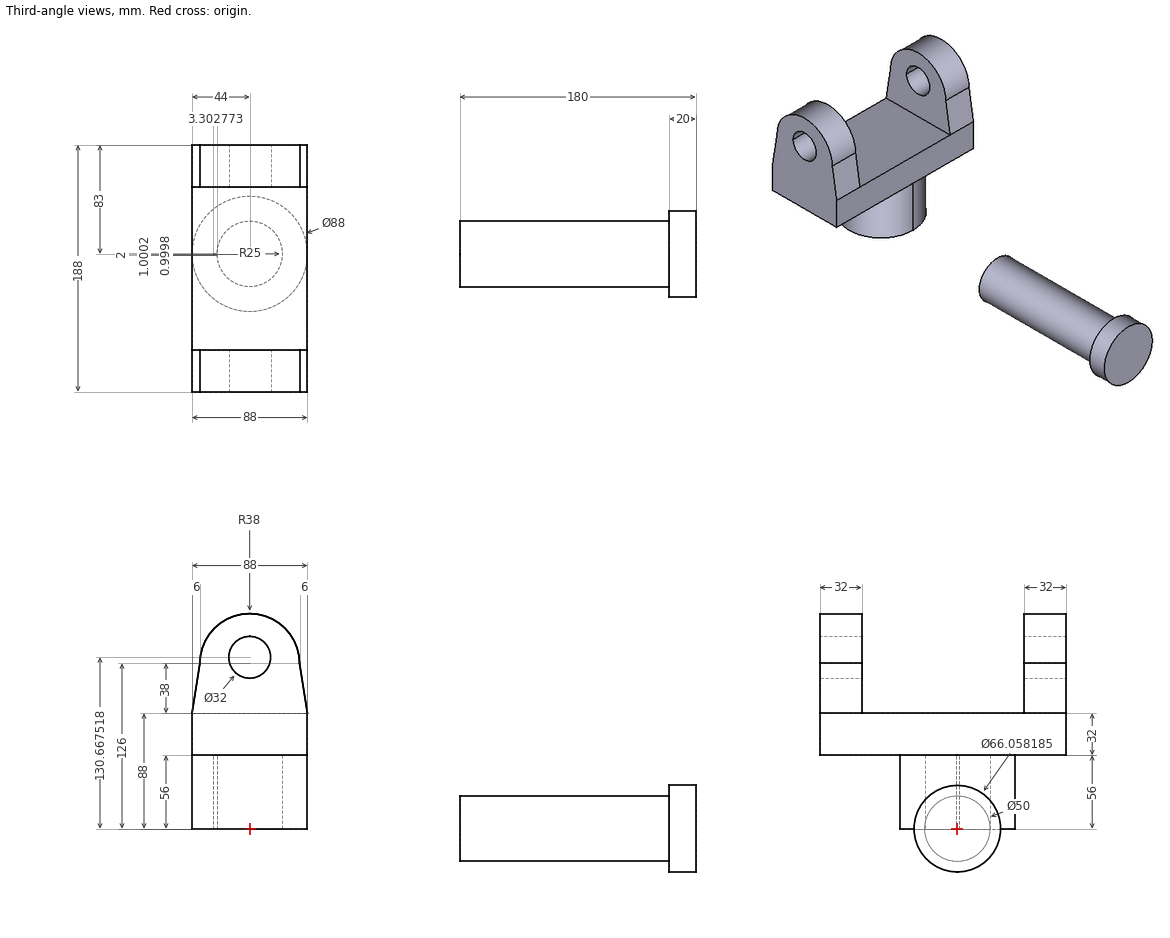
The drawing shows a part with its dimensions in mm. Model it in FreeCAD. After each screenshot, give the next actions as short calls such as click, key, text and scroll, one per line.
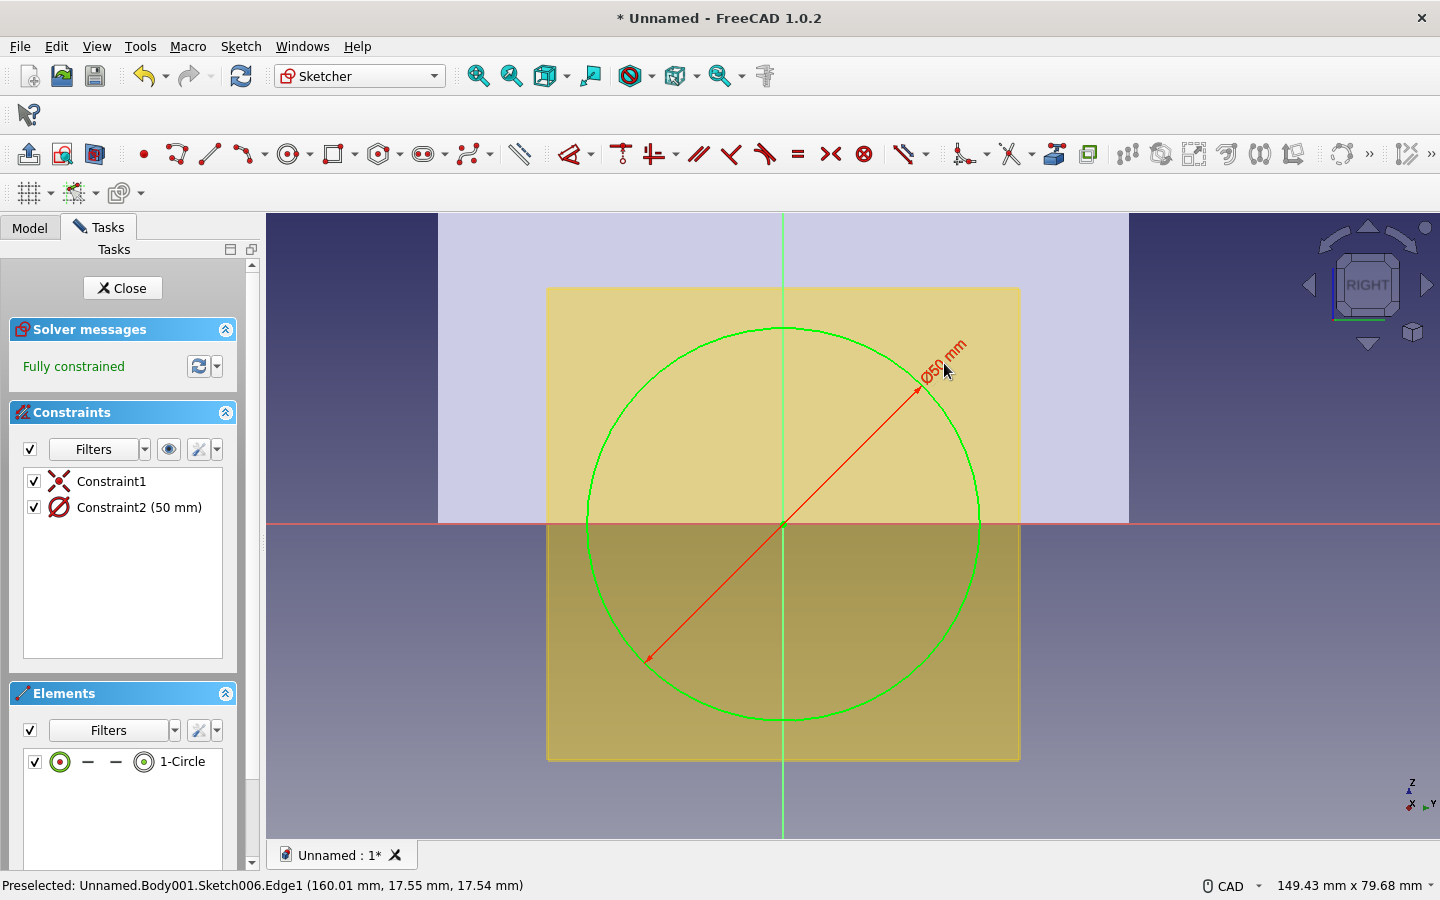
click(123, 288)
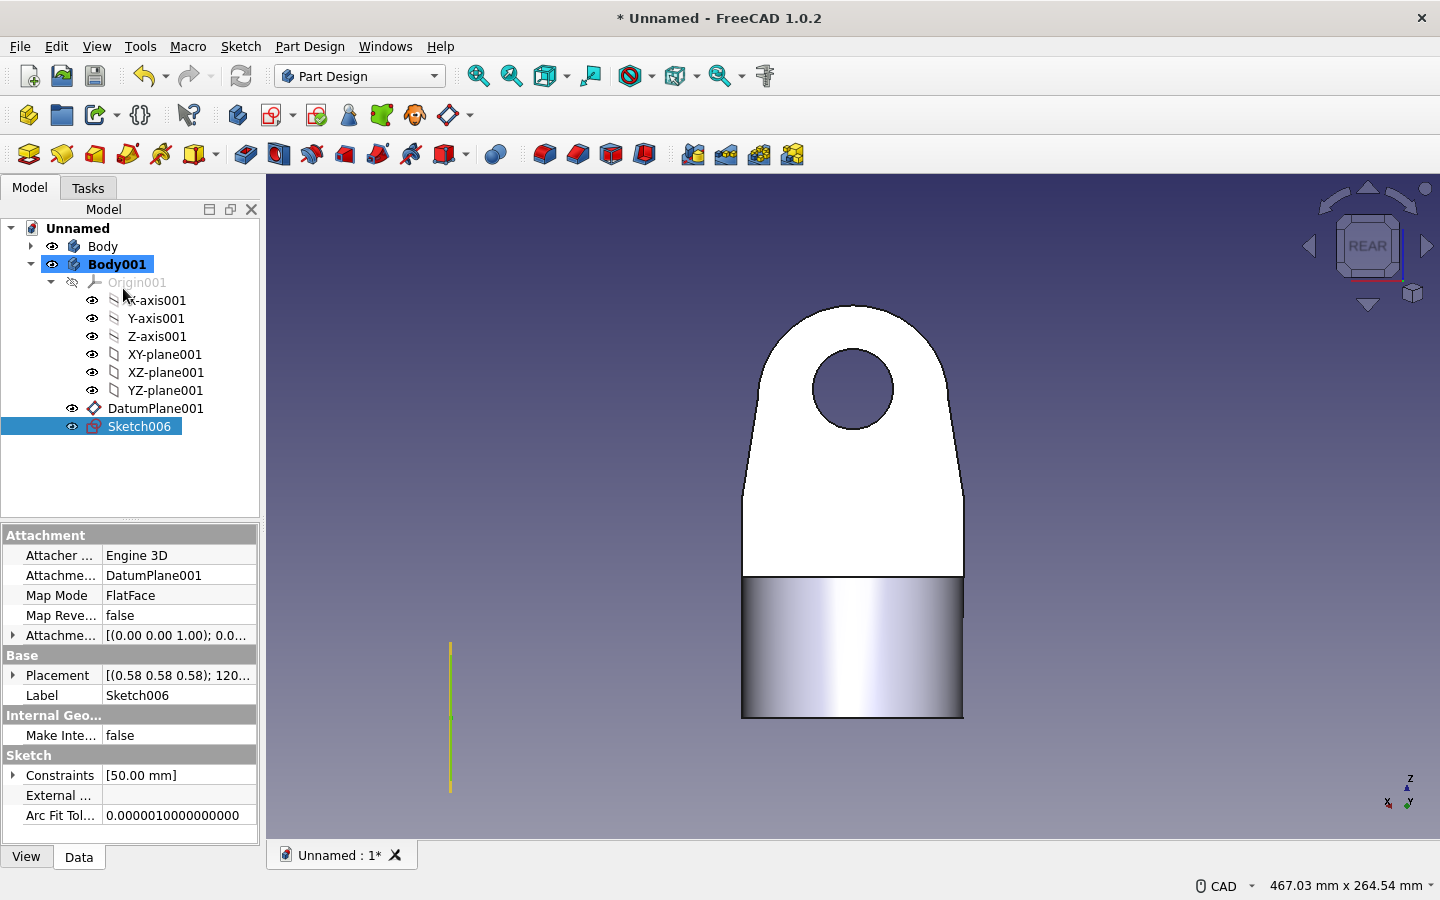
click(29, 154)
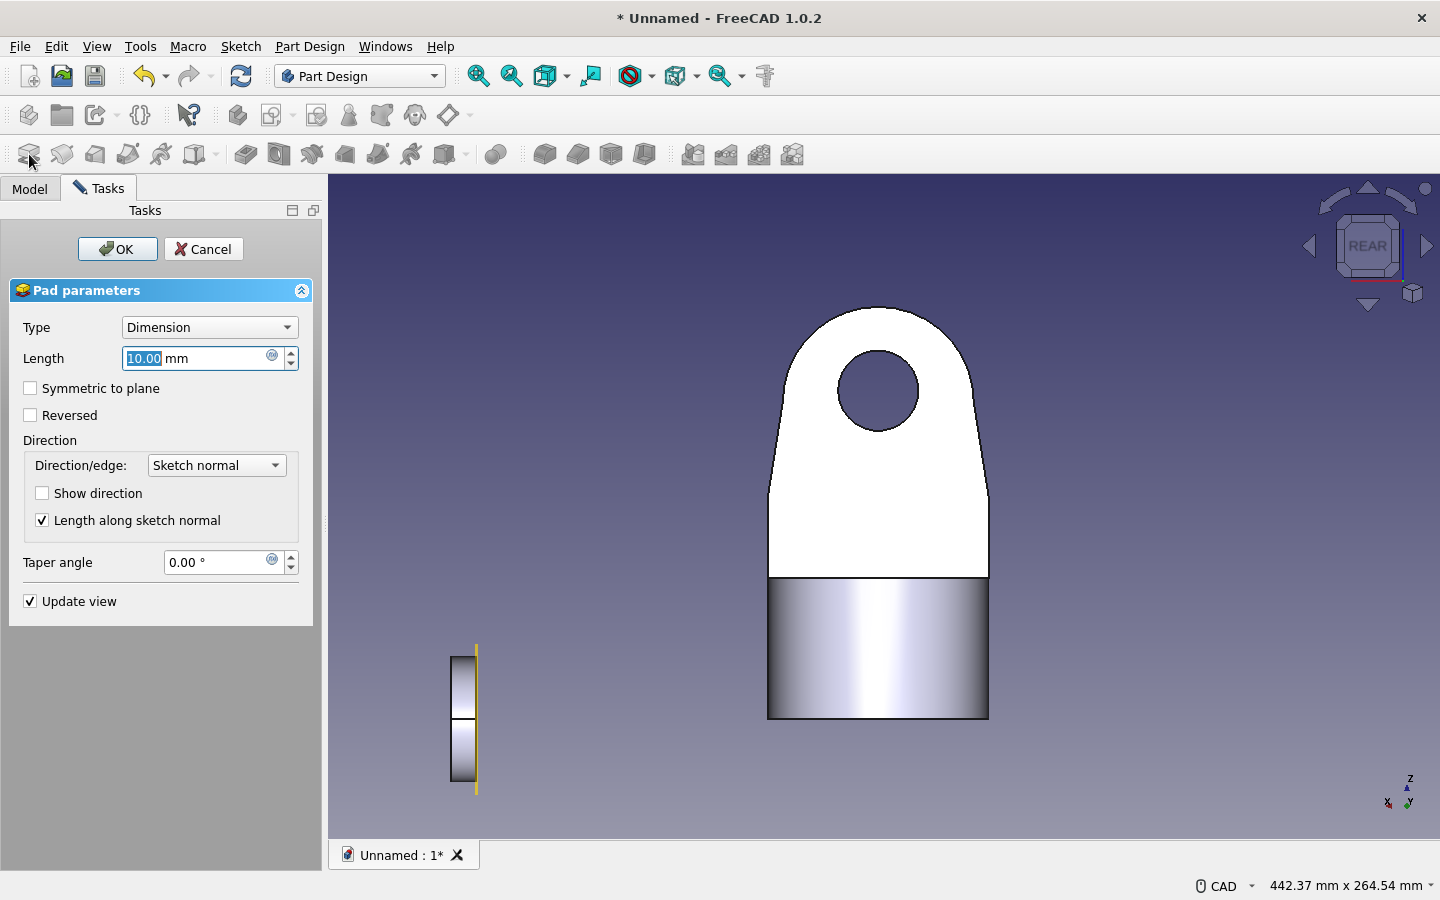
text(180)
key(Tab)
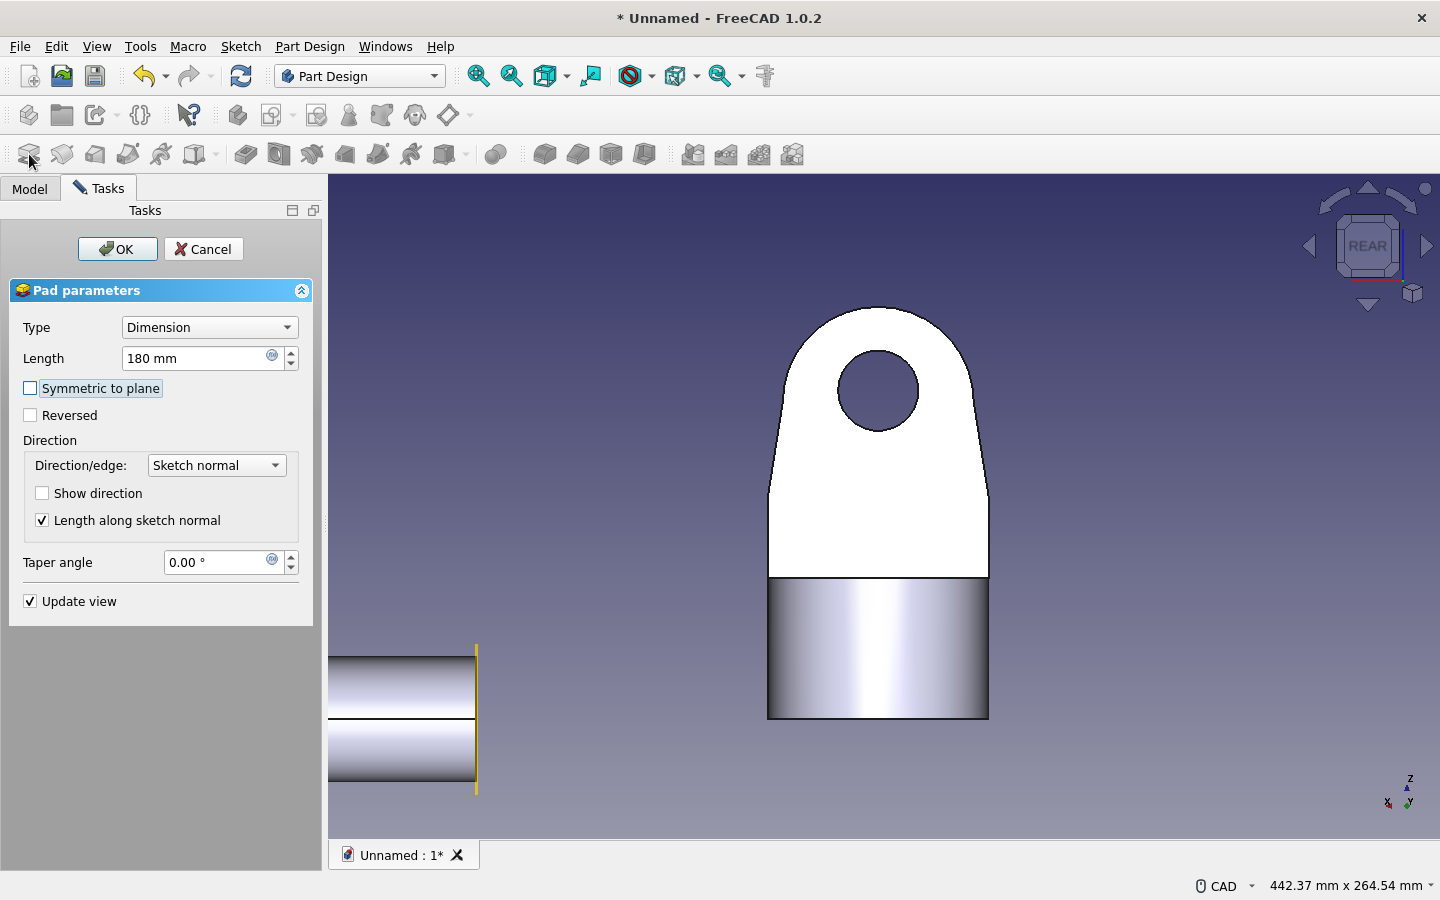
click(118, 249)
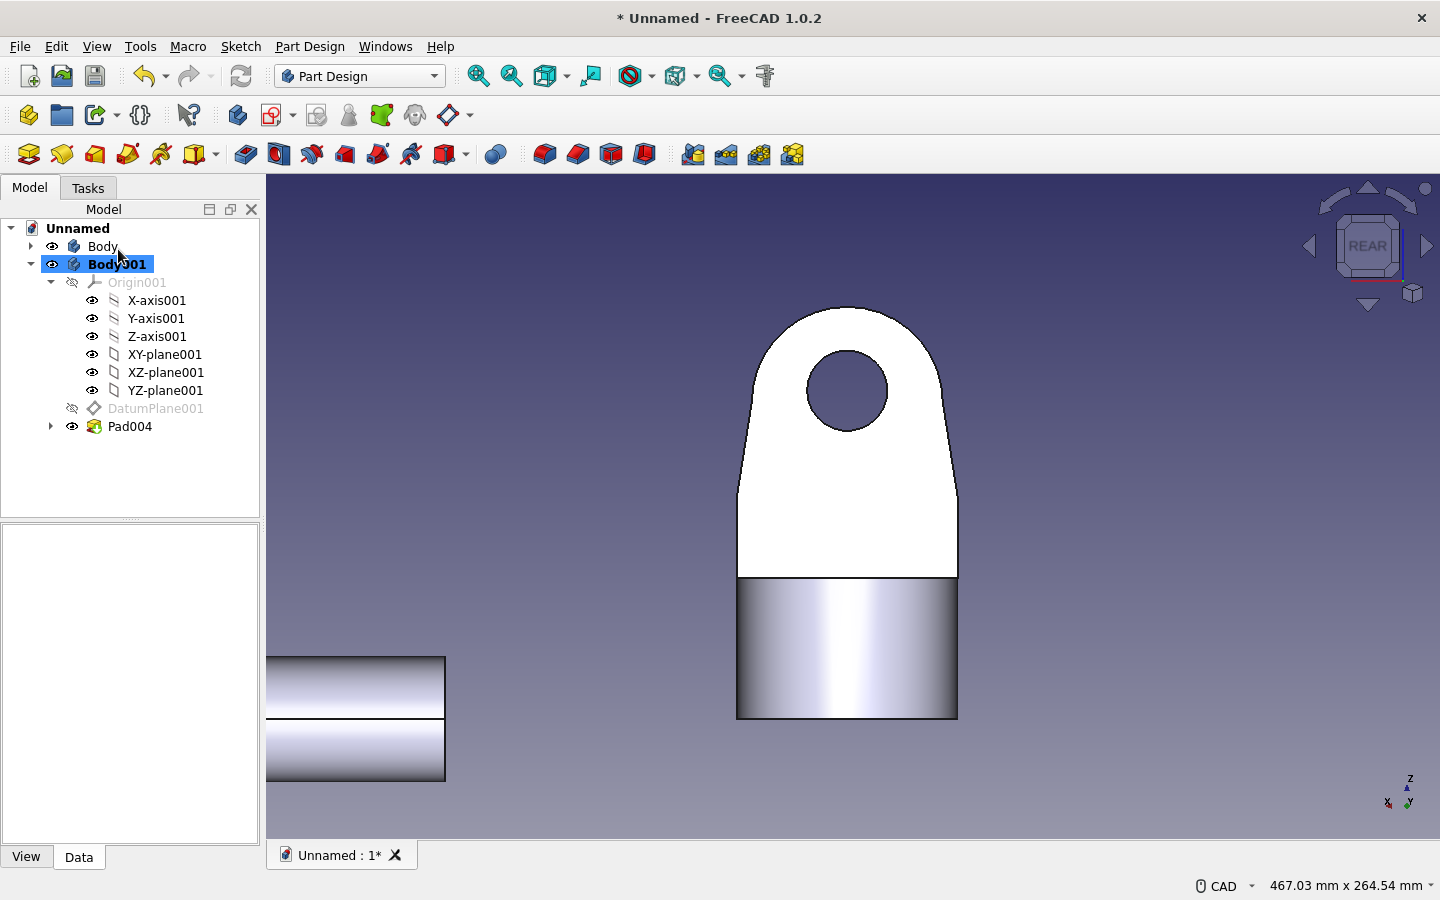
key(v)
key(f)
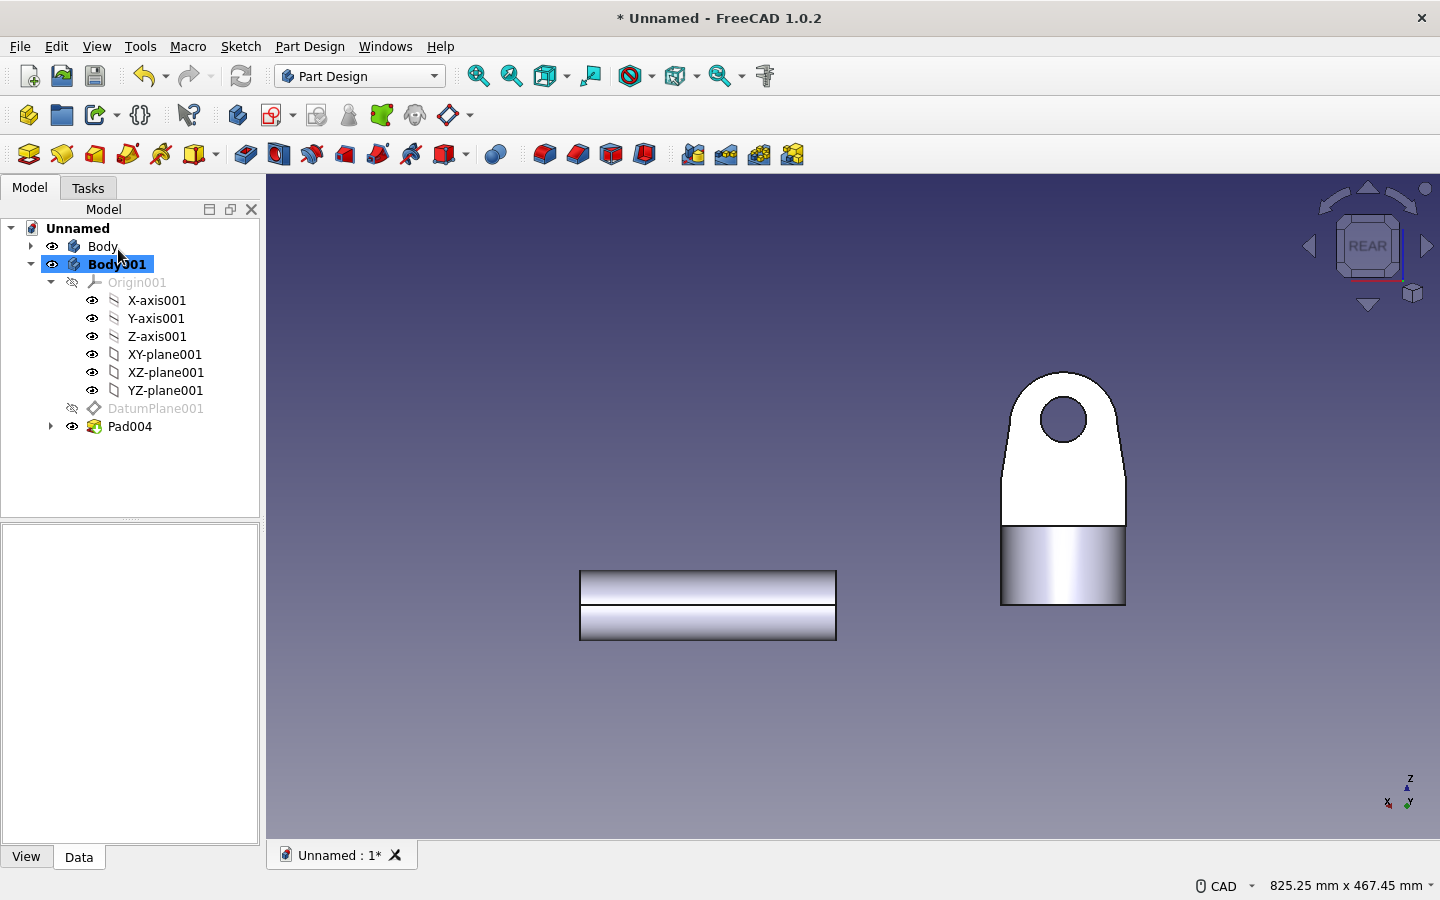
key(0)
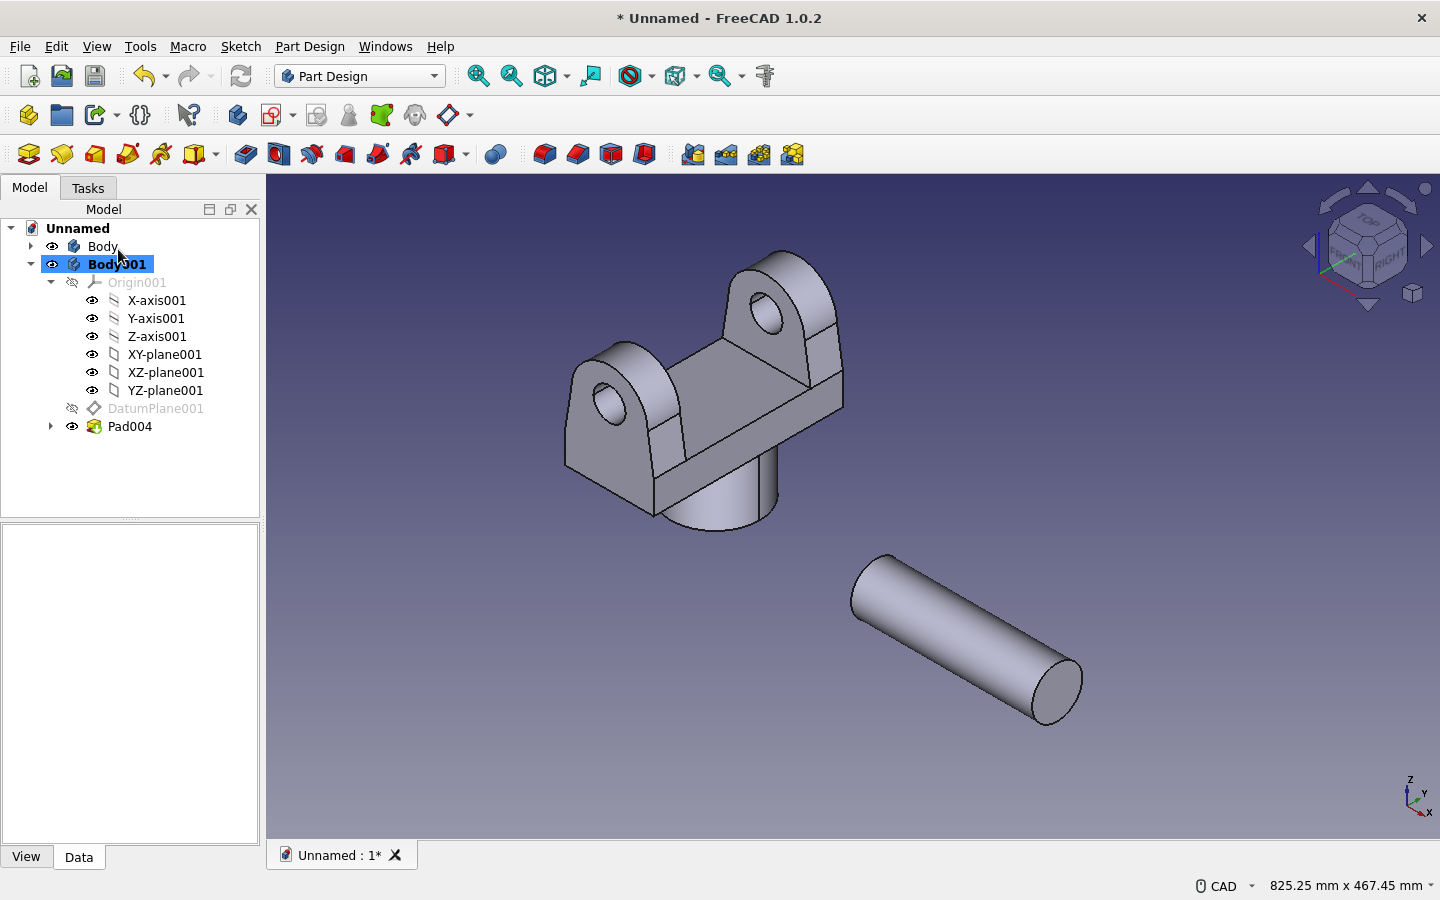
key(v)
key(f)